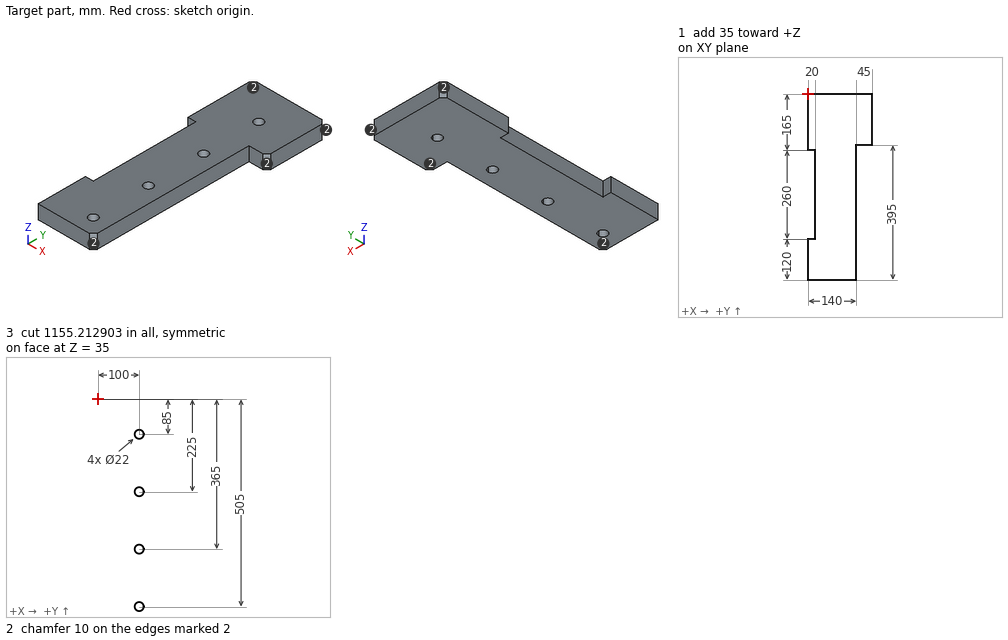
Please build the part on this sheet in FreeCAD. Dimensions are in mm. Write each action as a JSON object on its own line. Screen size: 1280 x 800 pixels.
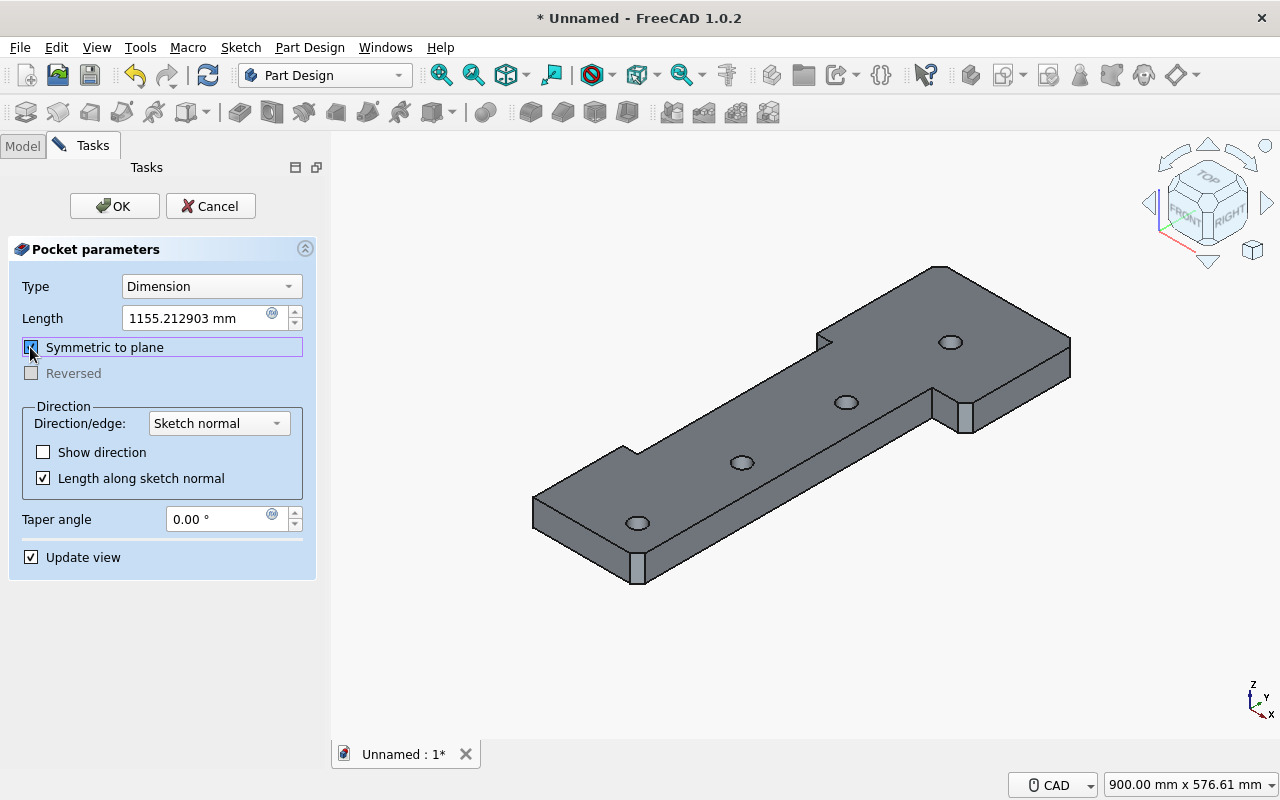
{"action": "left_click", "coordinate": [115, 206]}